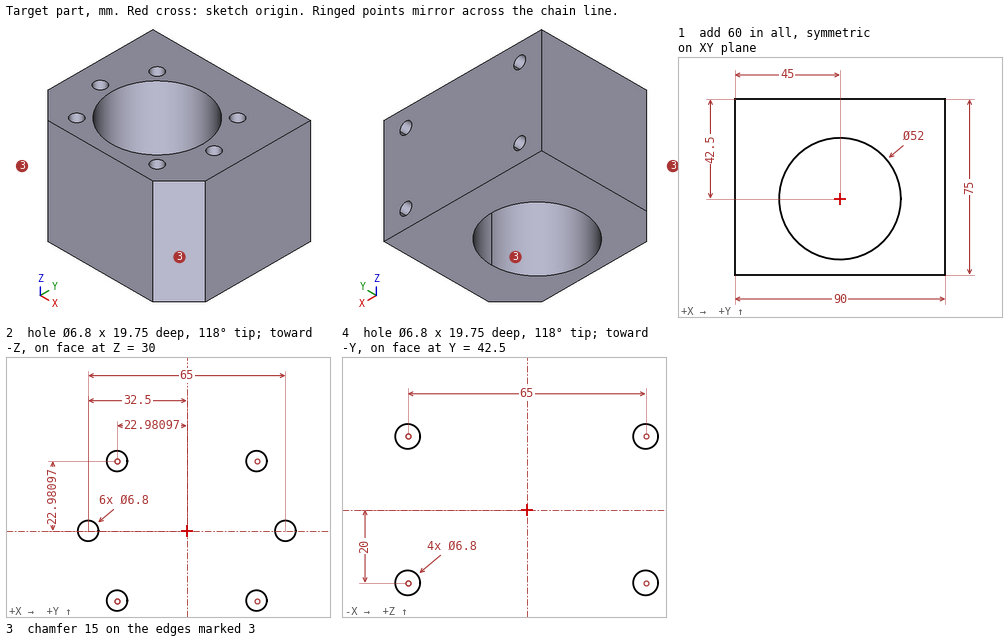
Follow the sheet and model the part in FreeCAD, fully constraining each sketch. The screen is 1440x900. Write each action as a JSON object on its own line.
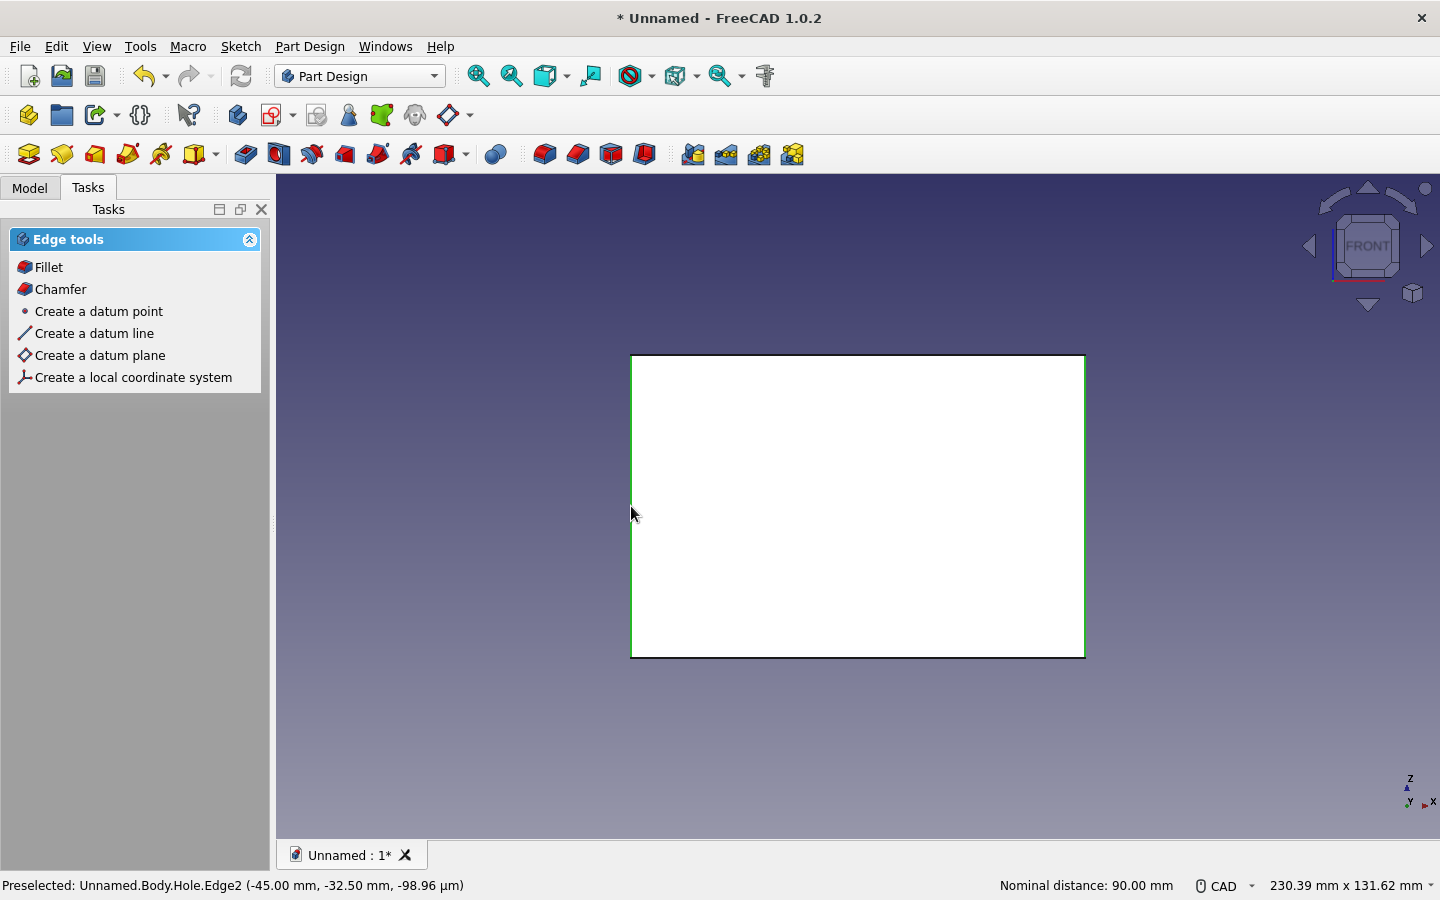
{"action": "left_click", "coordinate": [578, 154]}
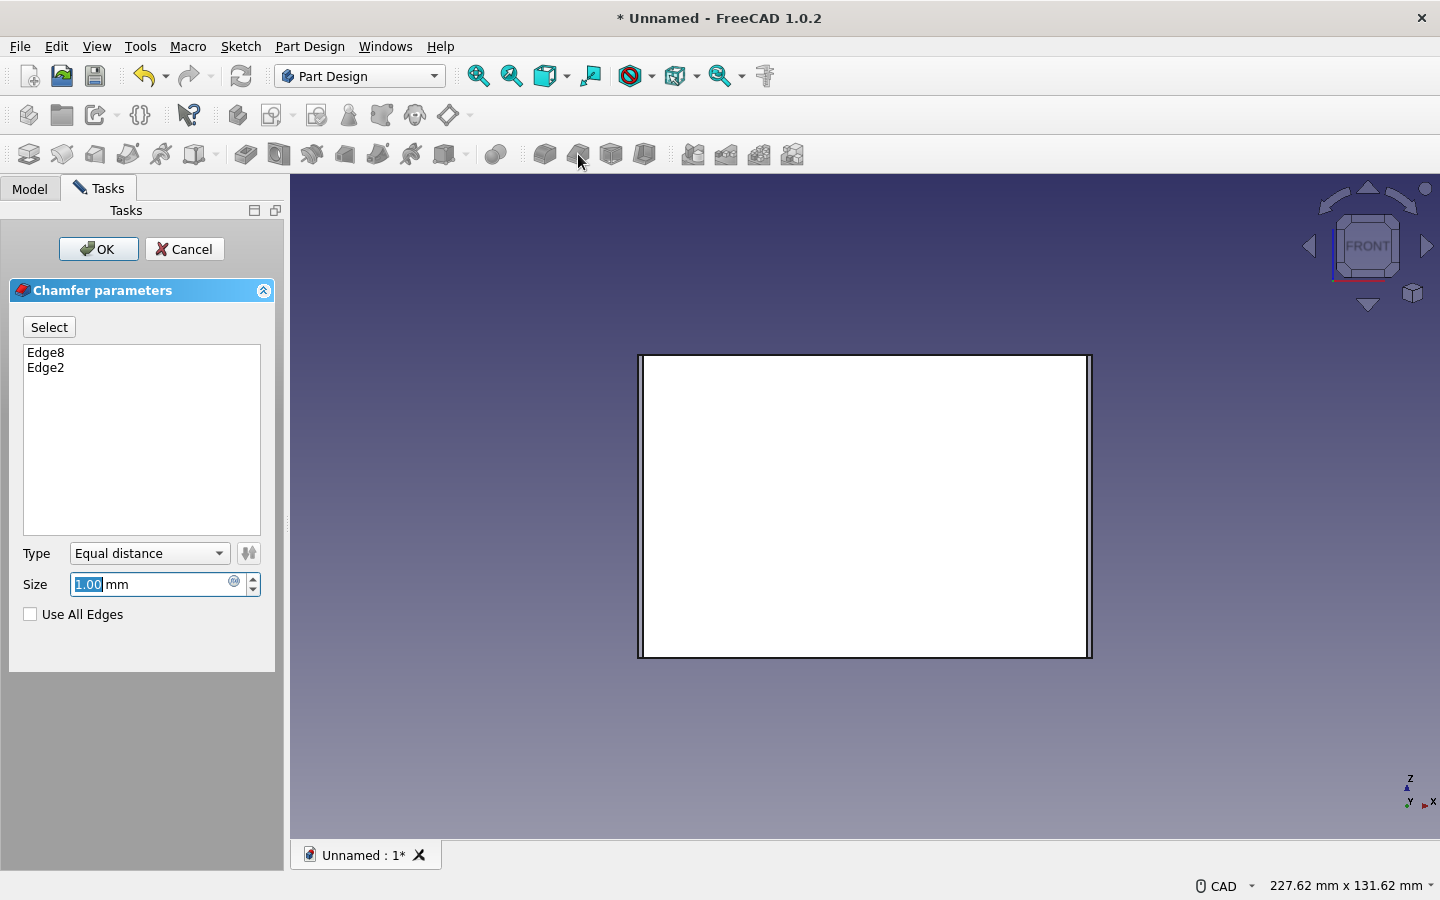
{"action": "type", "text": "15"}
{"action": "key", "text": "Tab"}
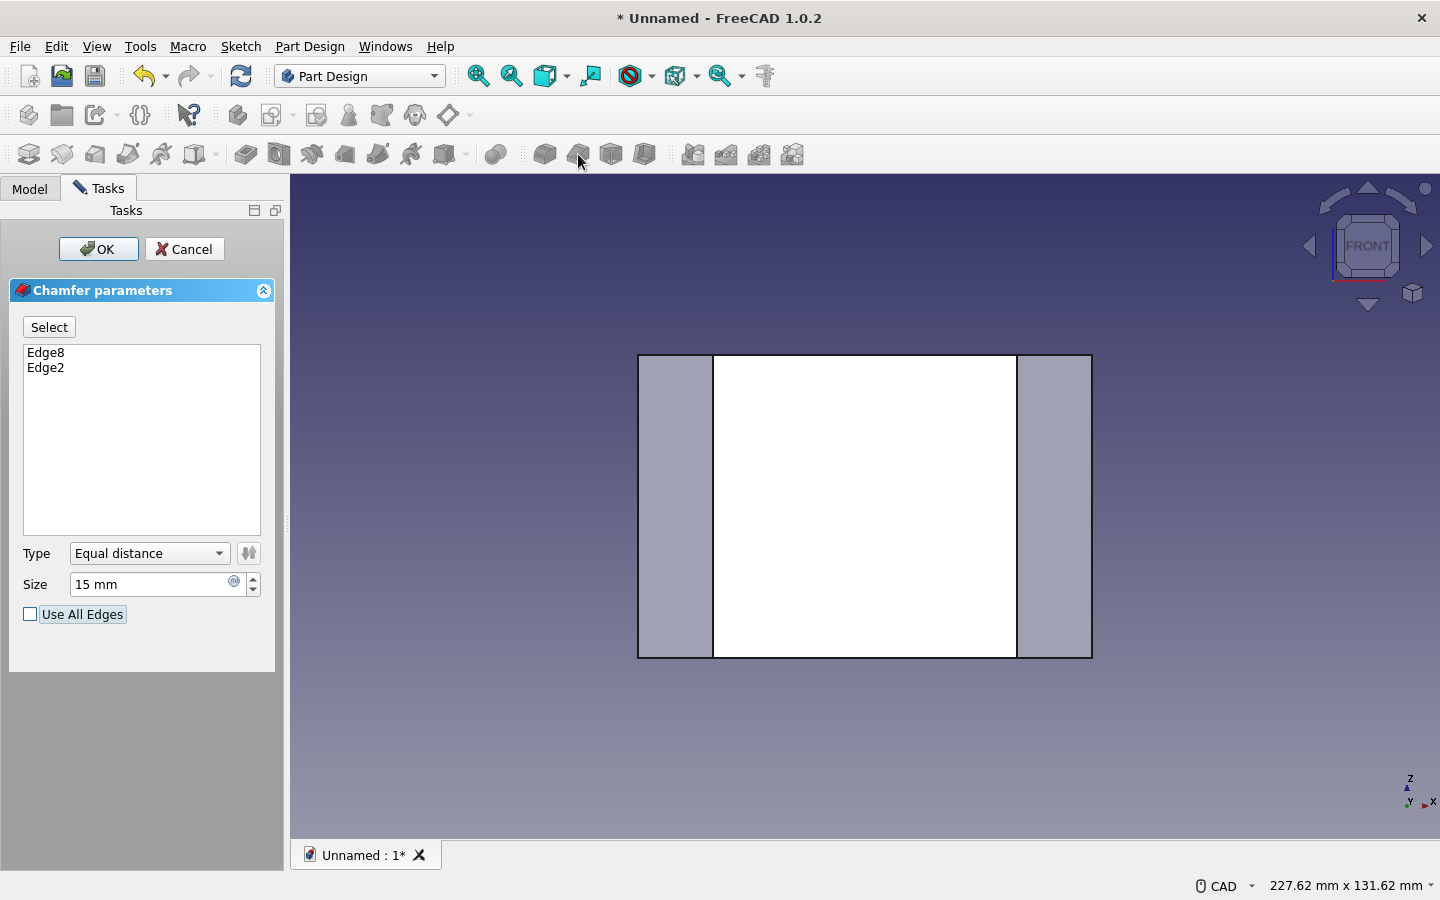
{"action": "left_click", "coordinate": [99, 249]}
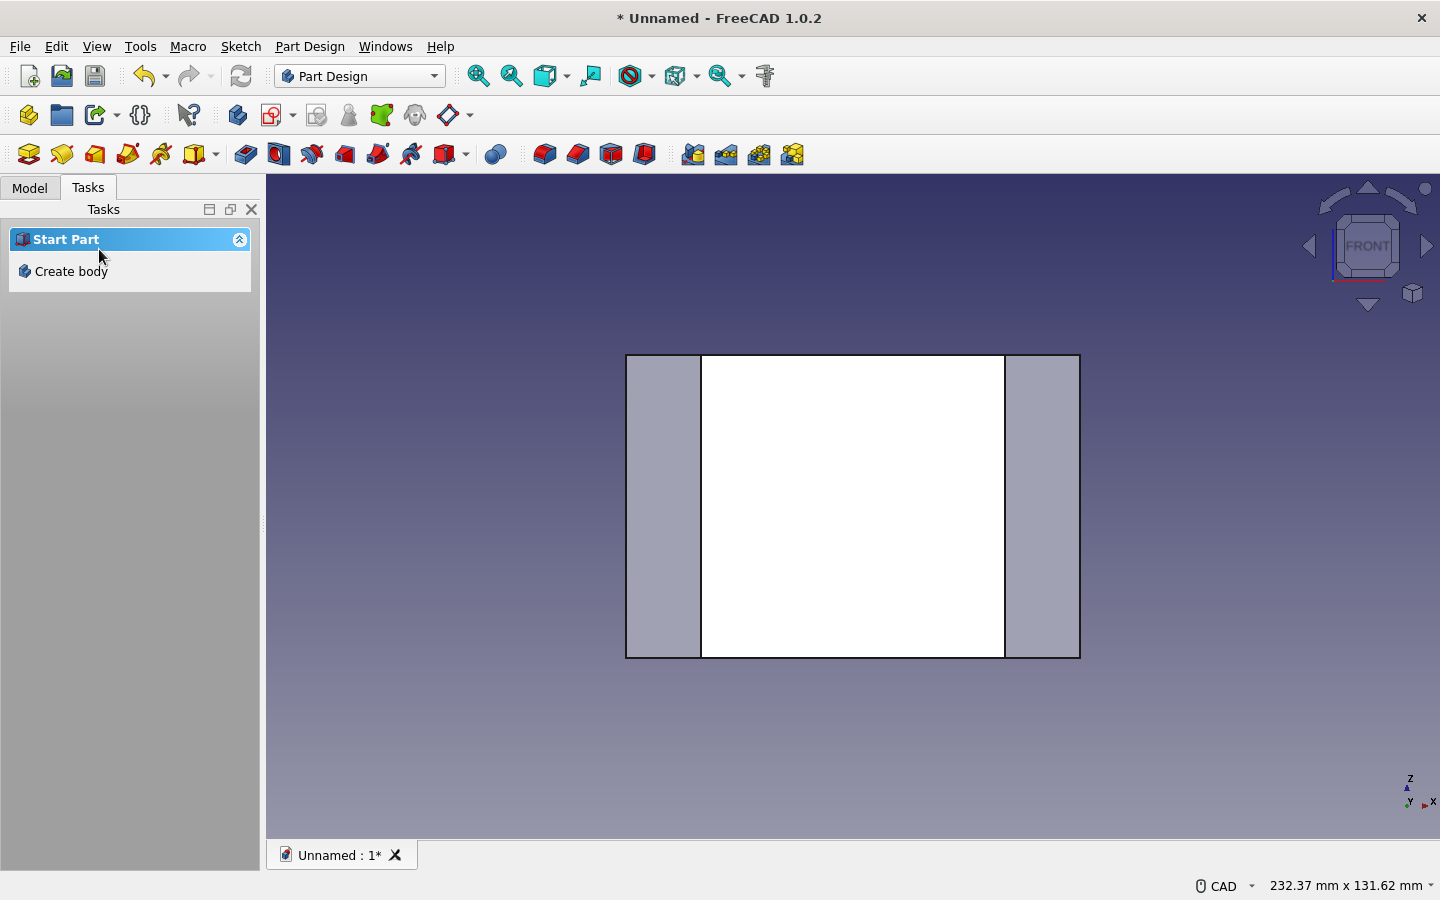
{"action": "key", "text": "4"}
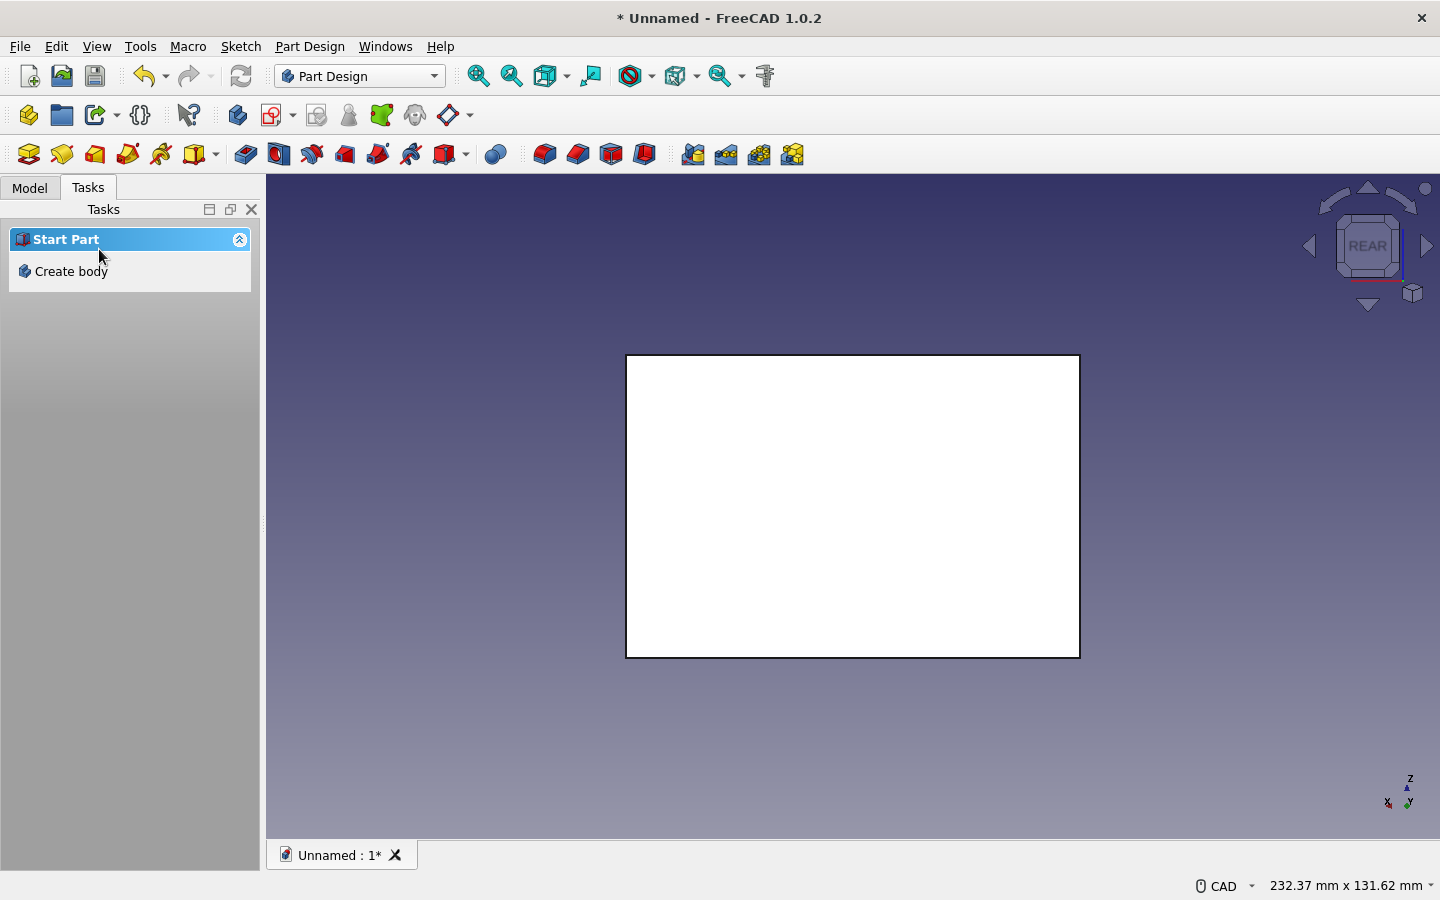
{"action": "left_click", "coordinate": [788, 506]}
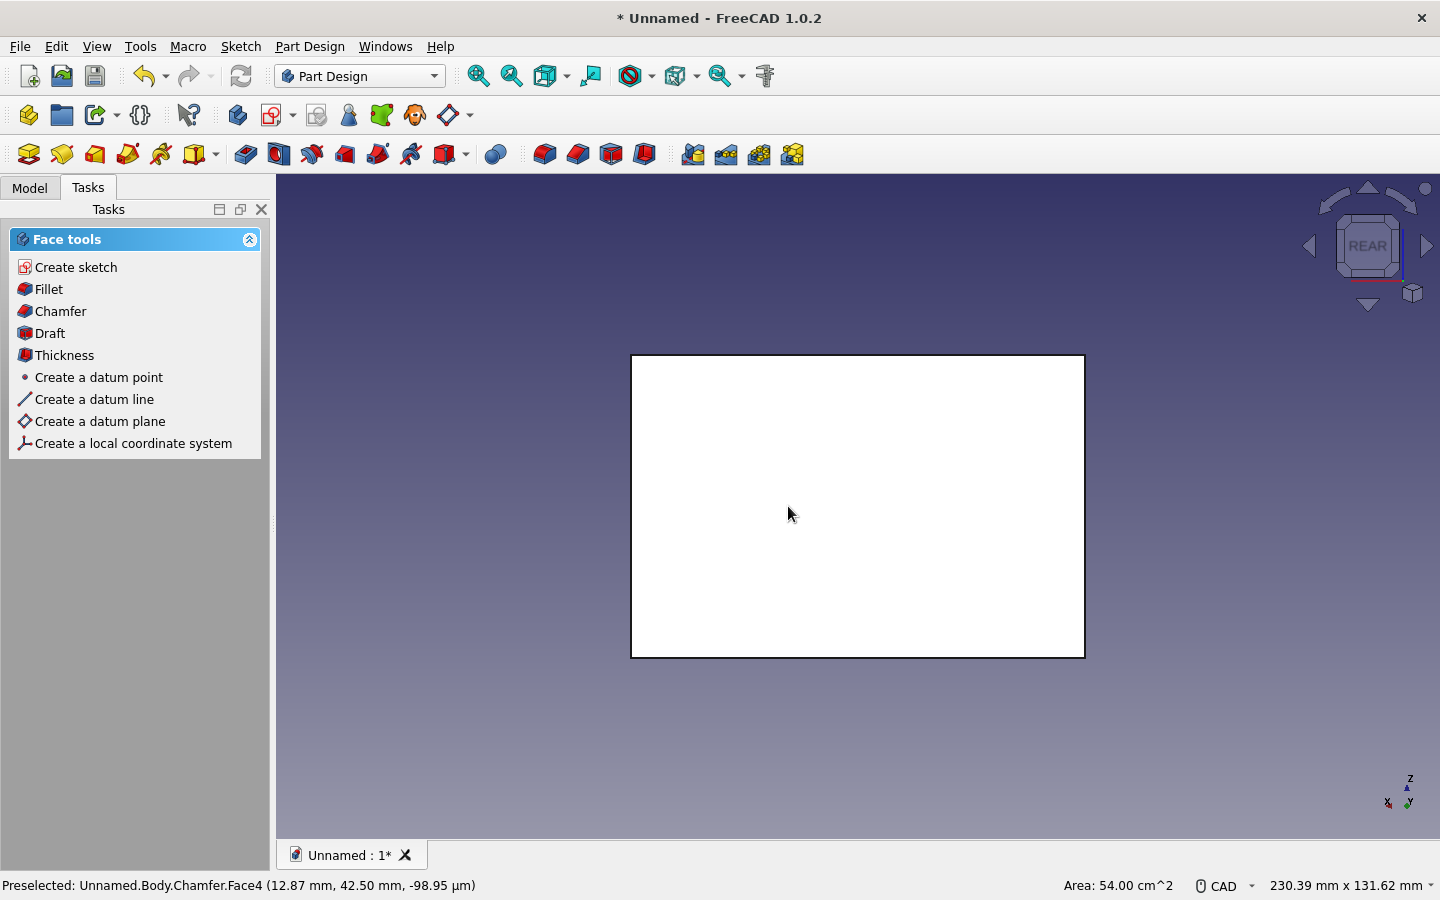
{"action": "left_click", "coordinate": [270, 116]}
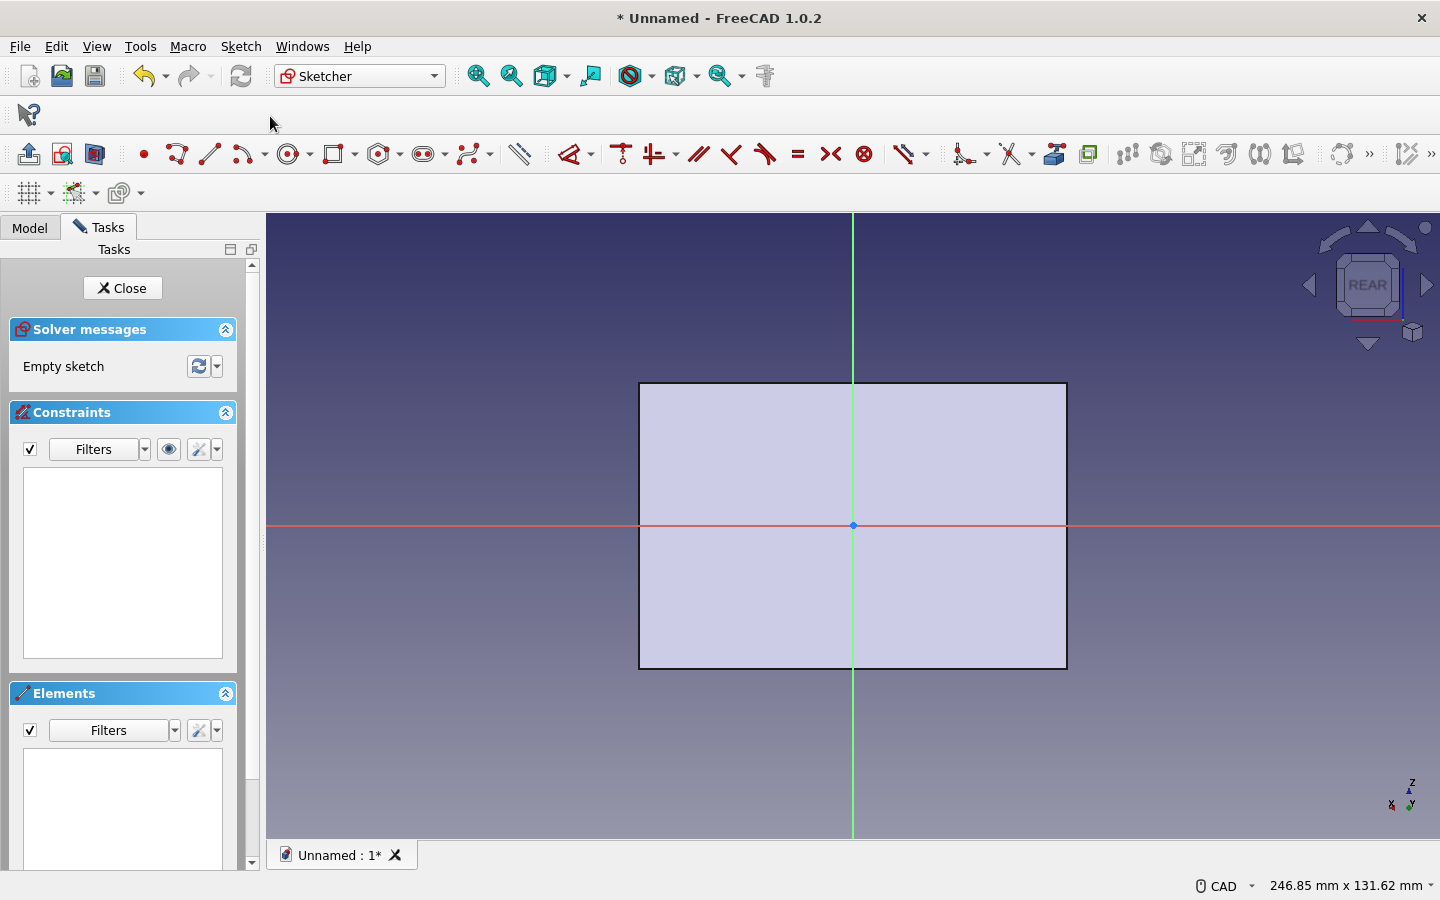
{"action": "scroll", "coordinate": [936, 526], "scroll_direction": "up", "scroll_amount": 3}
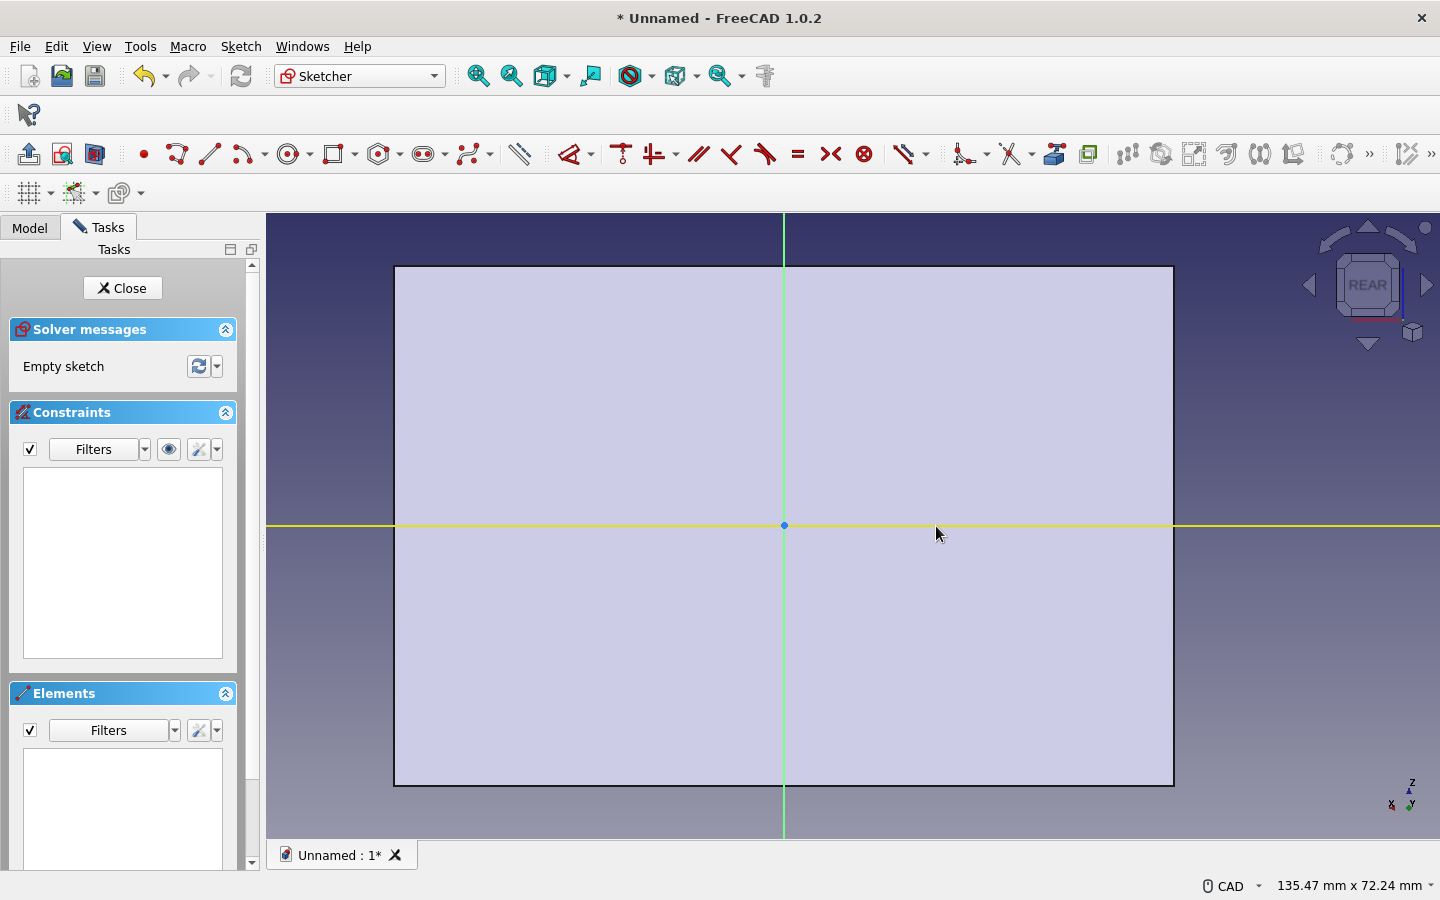
{"action": "left_click", "coordinate": [288, 154]}